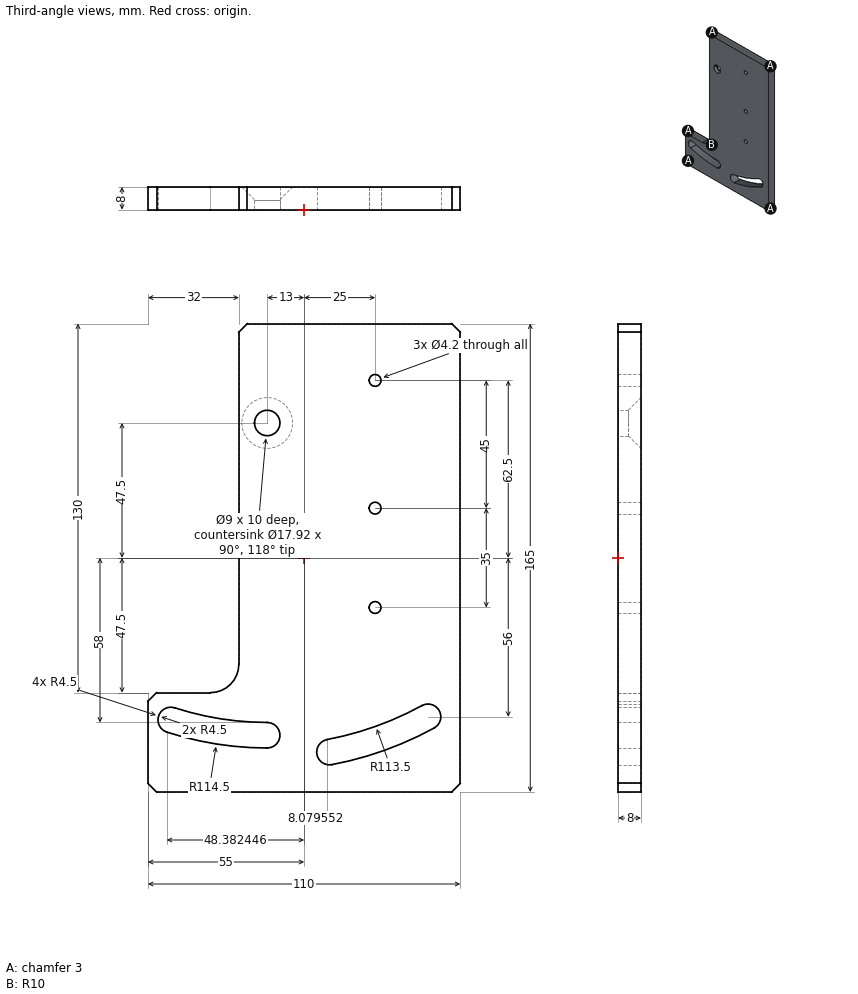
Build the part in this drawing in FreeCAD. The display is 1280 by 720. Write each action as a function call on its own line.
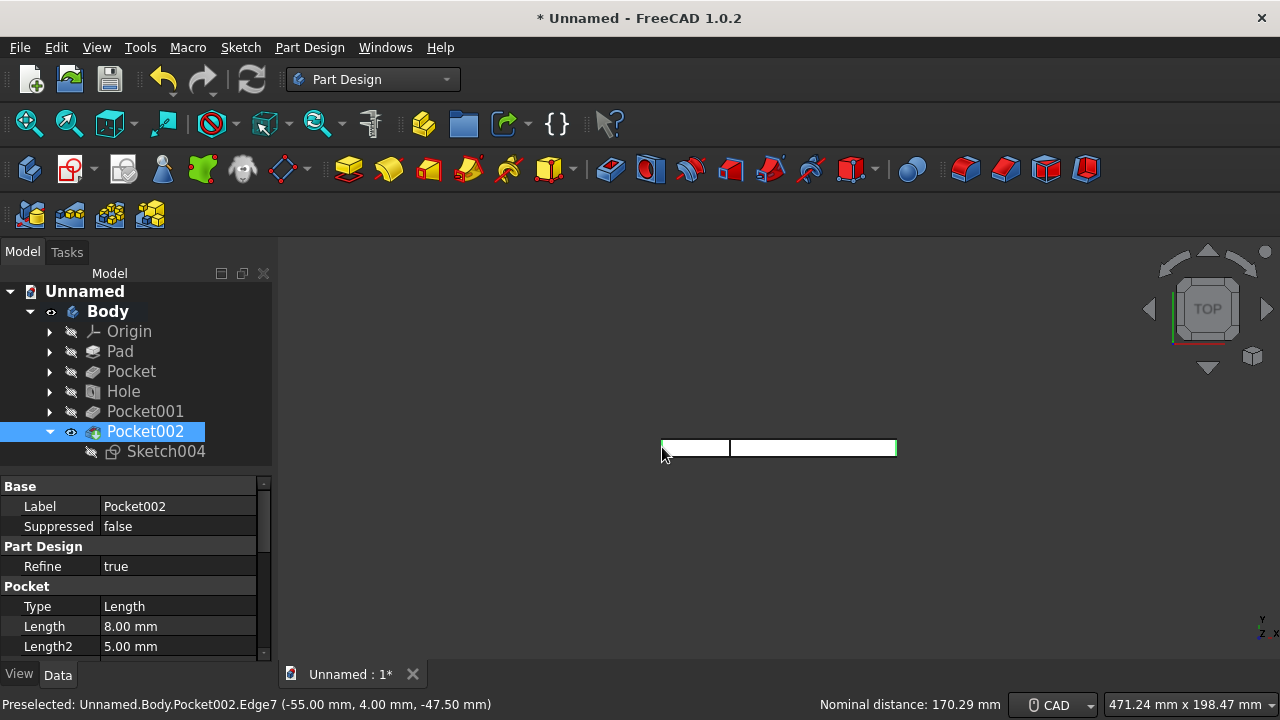
click(730, 447, ctrl)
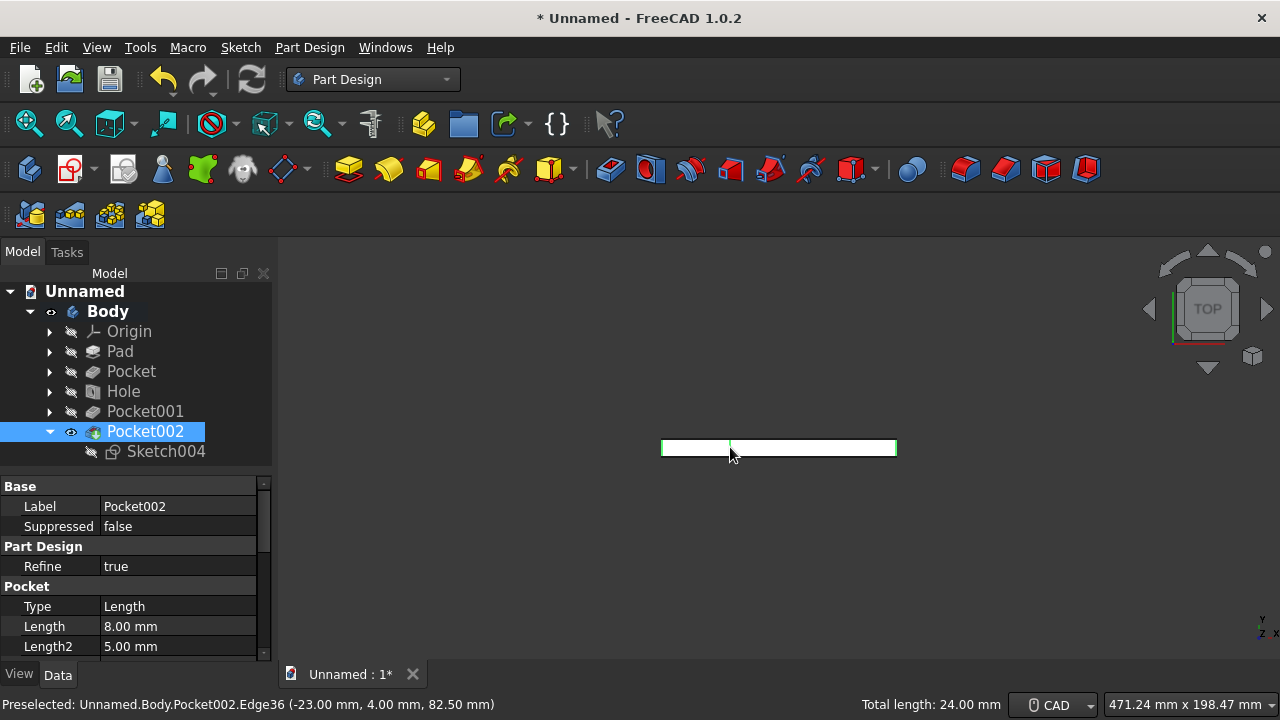
scroll(662, 447, up, 5)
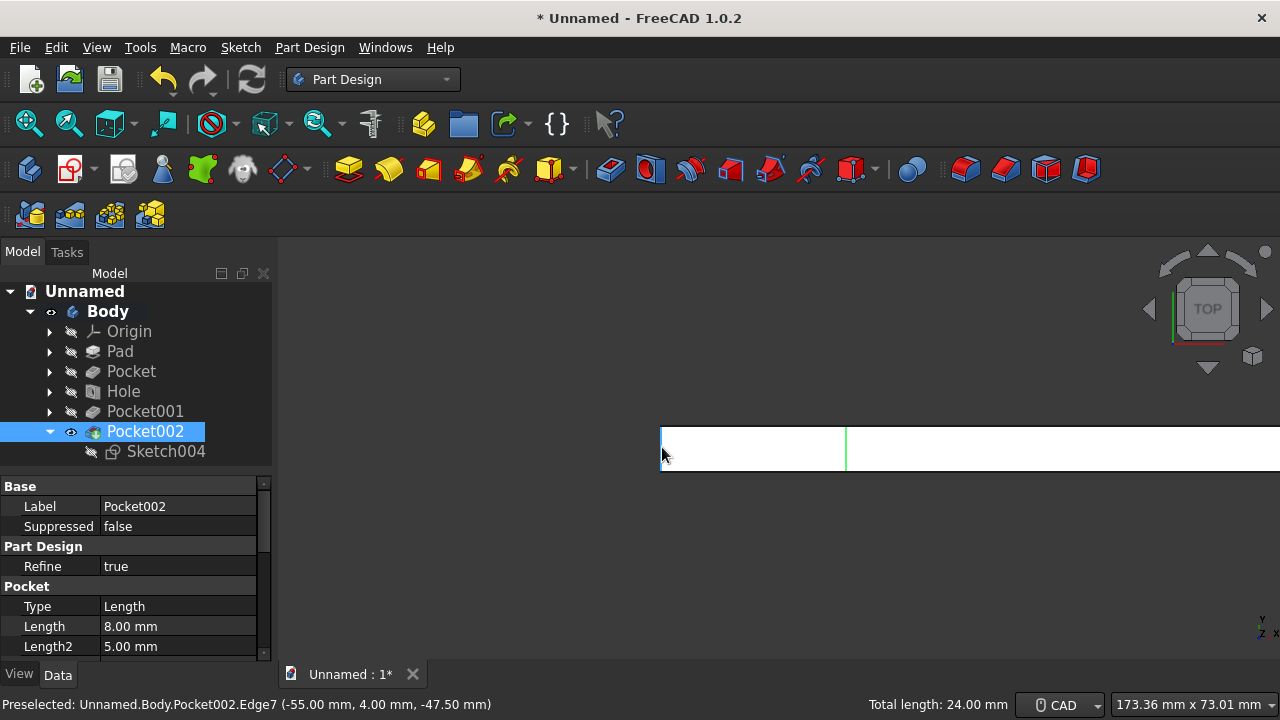
click(30, 124)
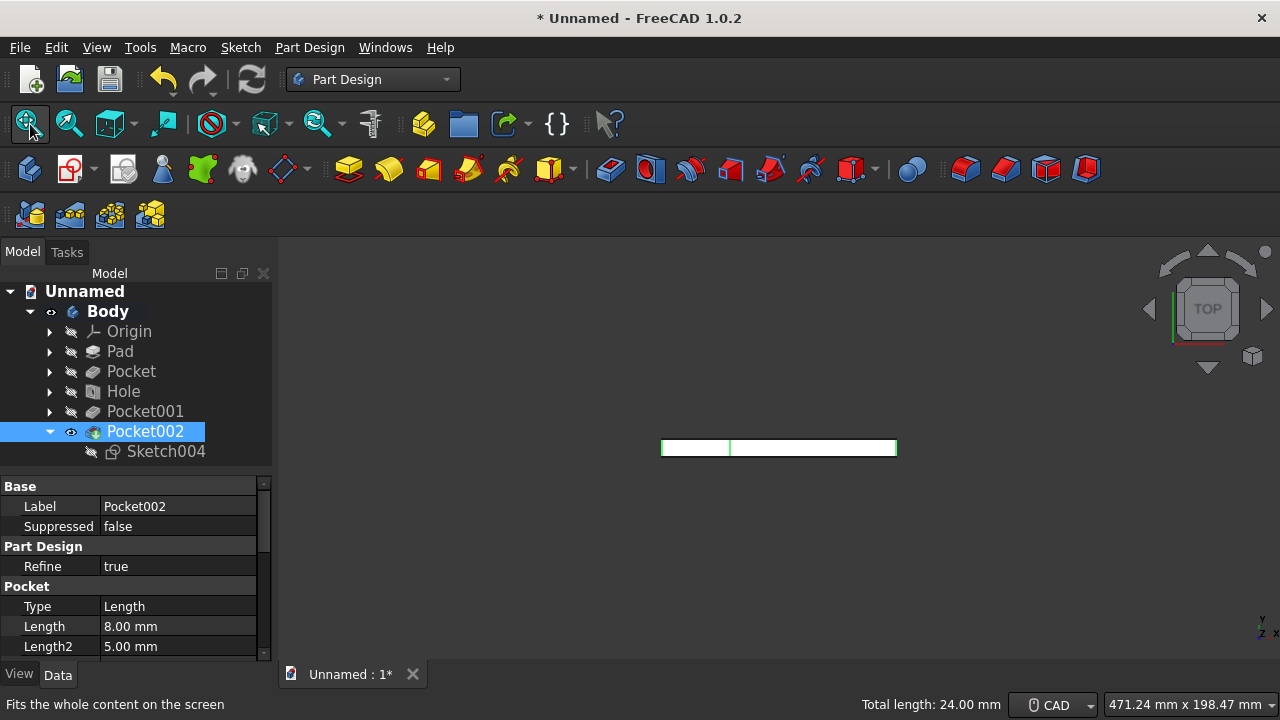
key(1)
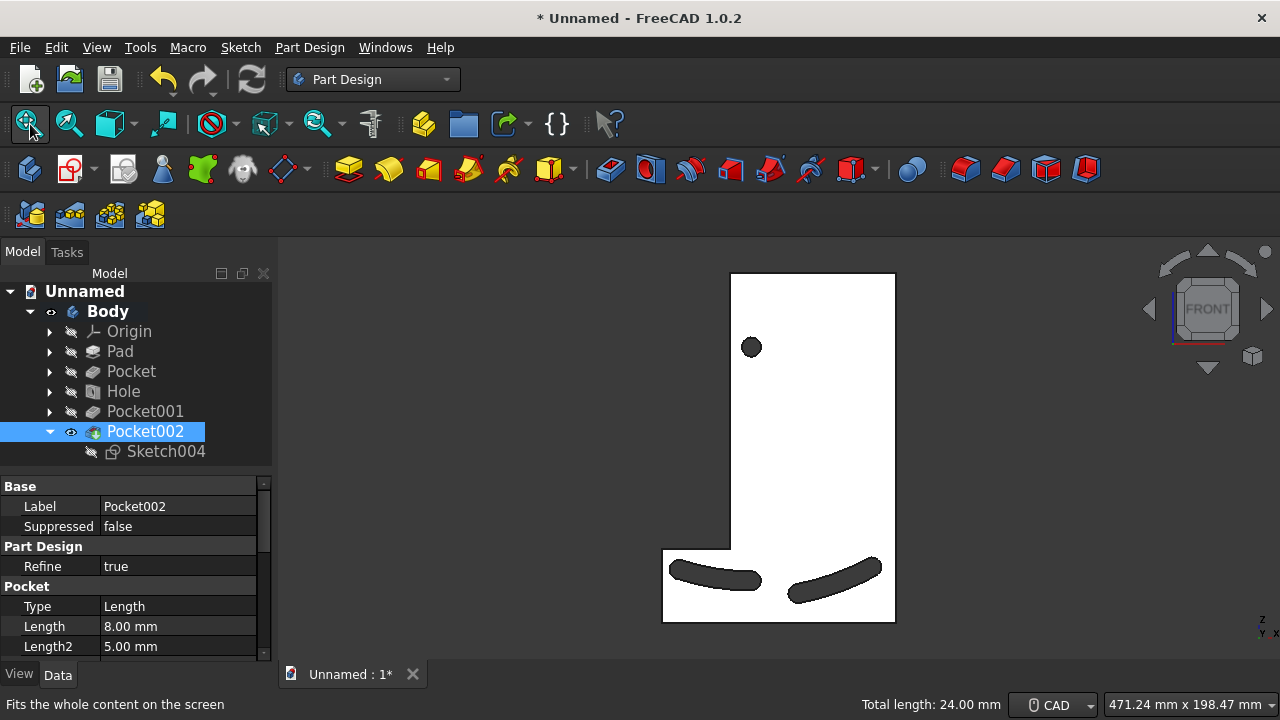
scroll(662, 622, up, 5)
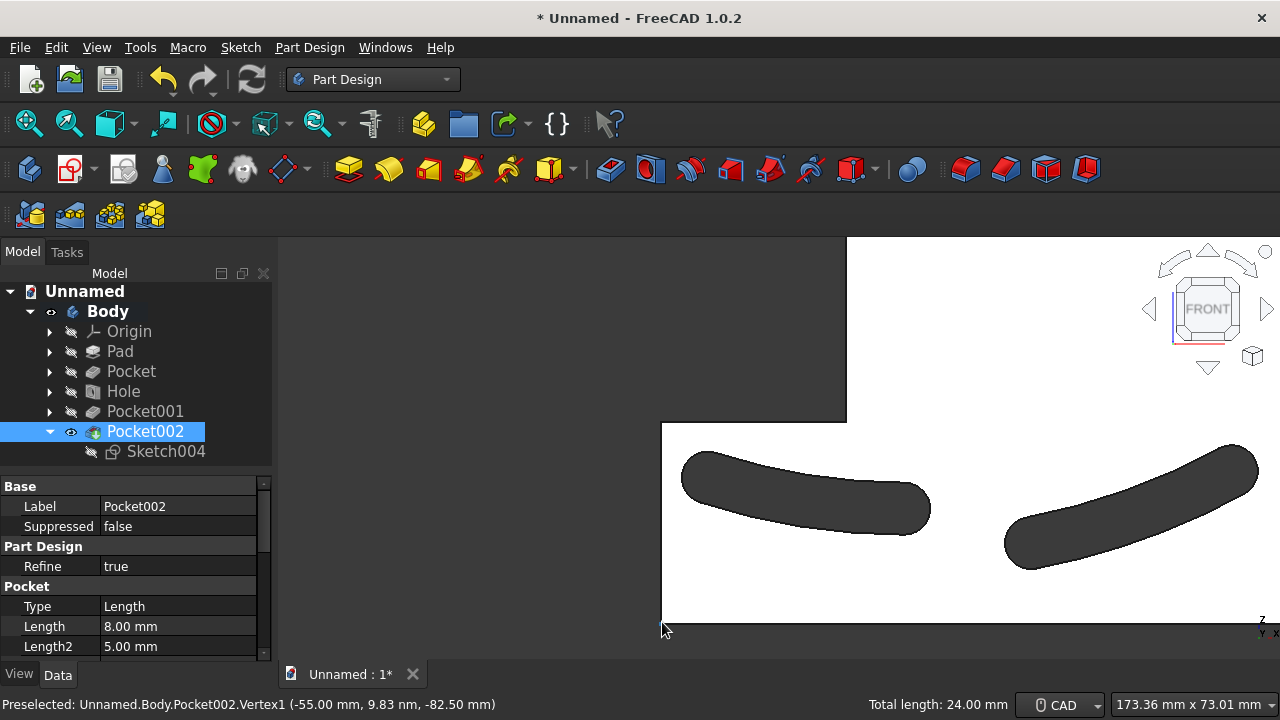
click(30, 124)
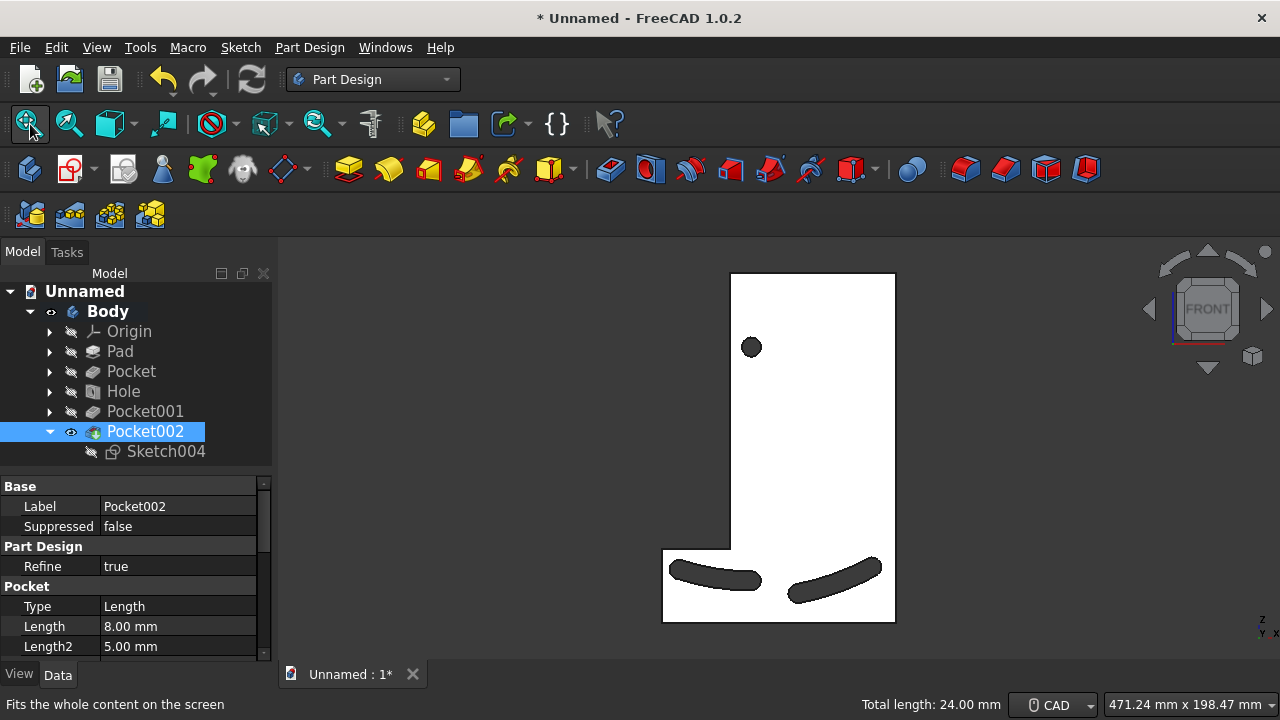
key(3)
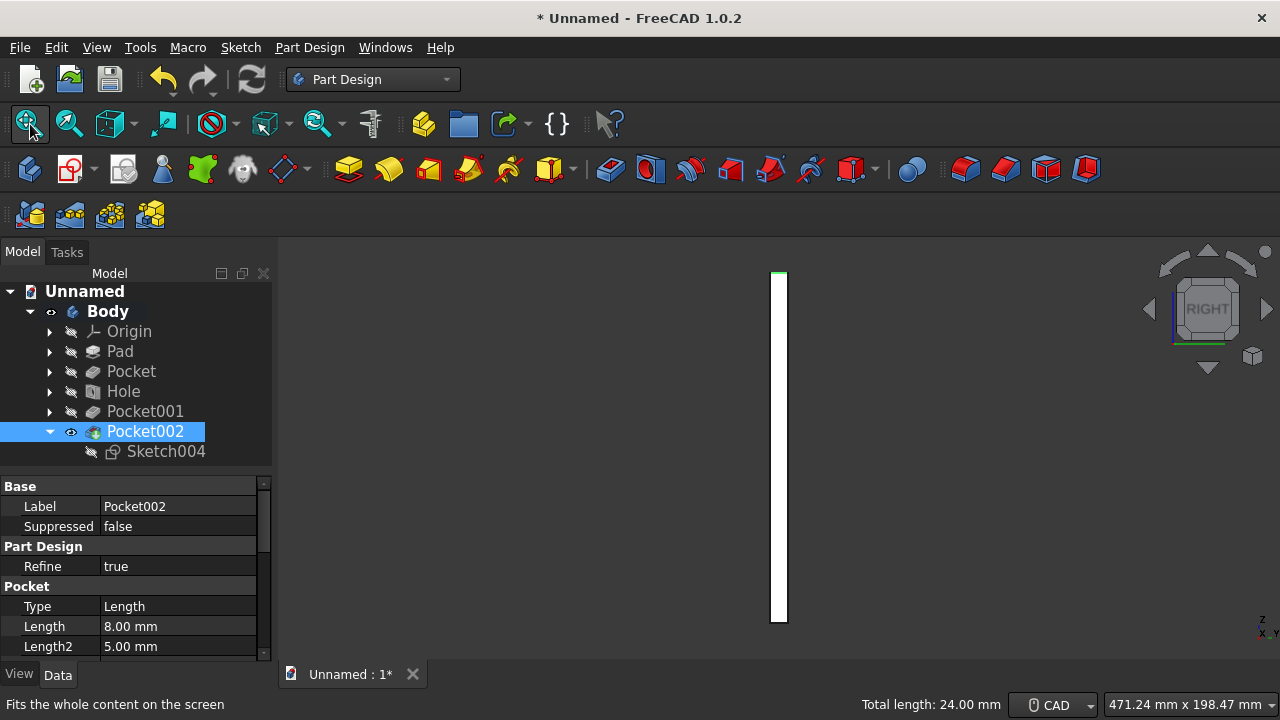
click(779, 622, ctrl)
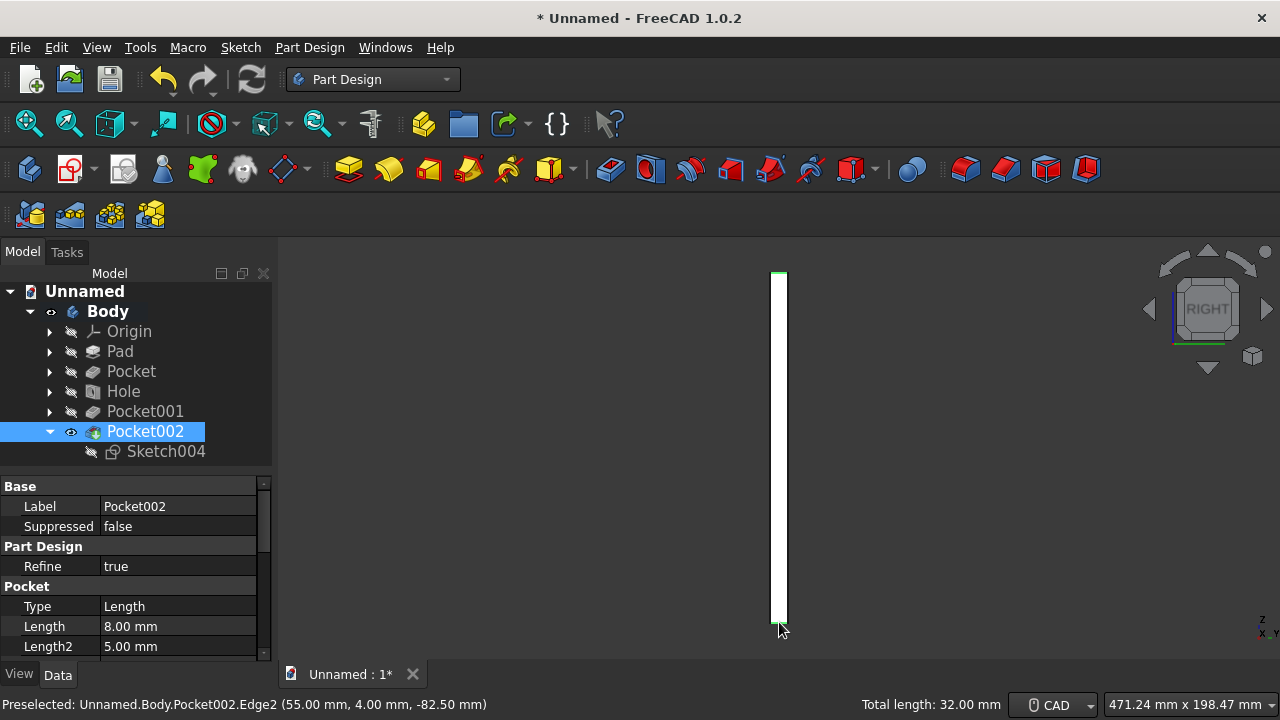
scroll(779, 622, up, 5)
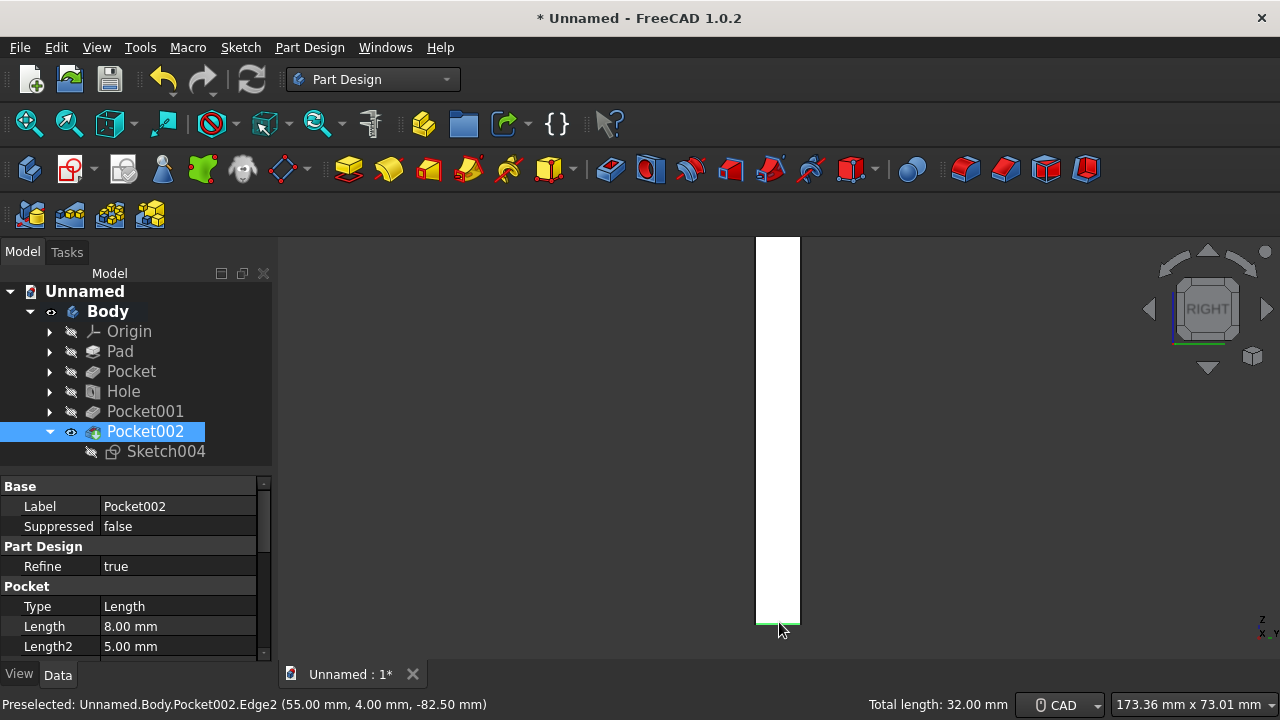
click(30, 124)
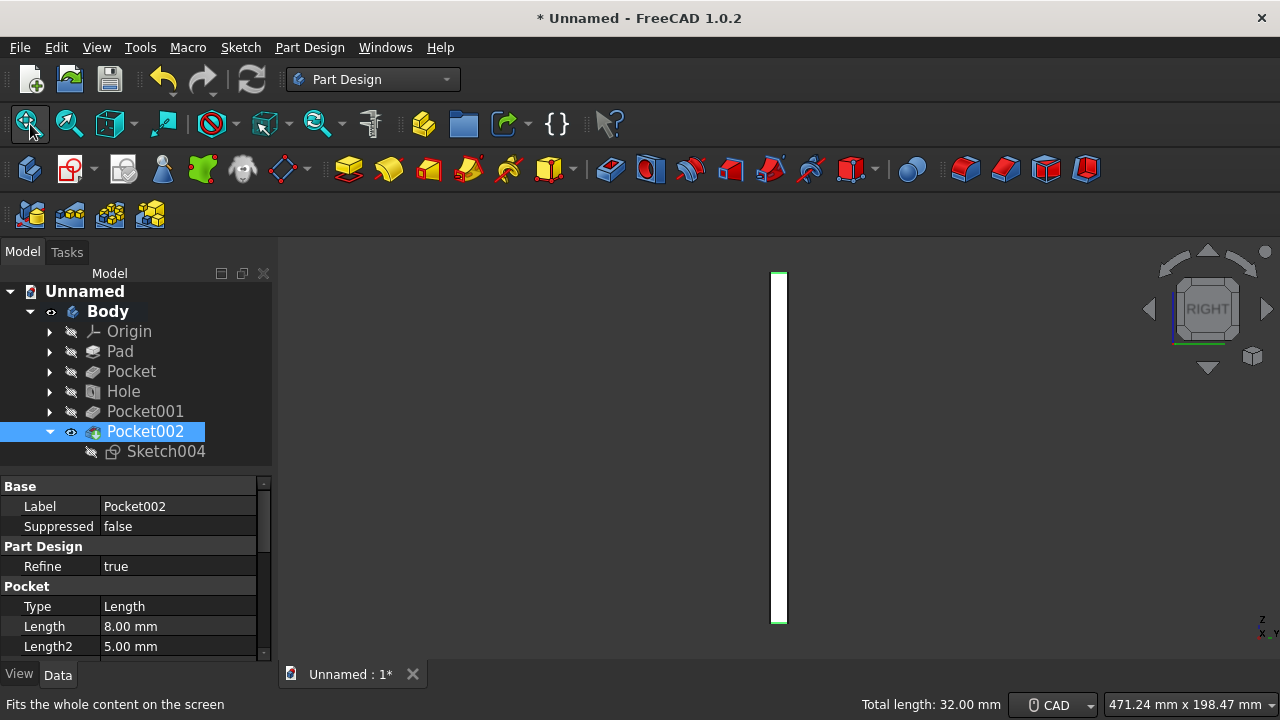
key(5)